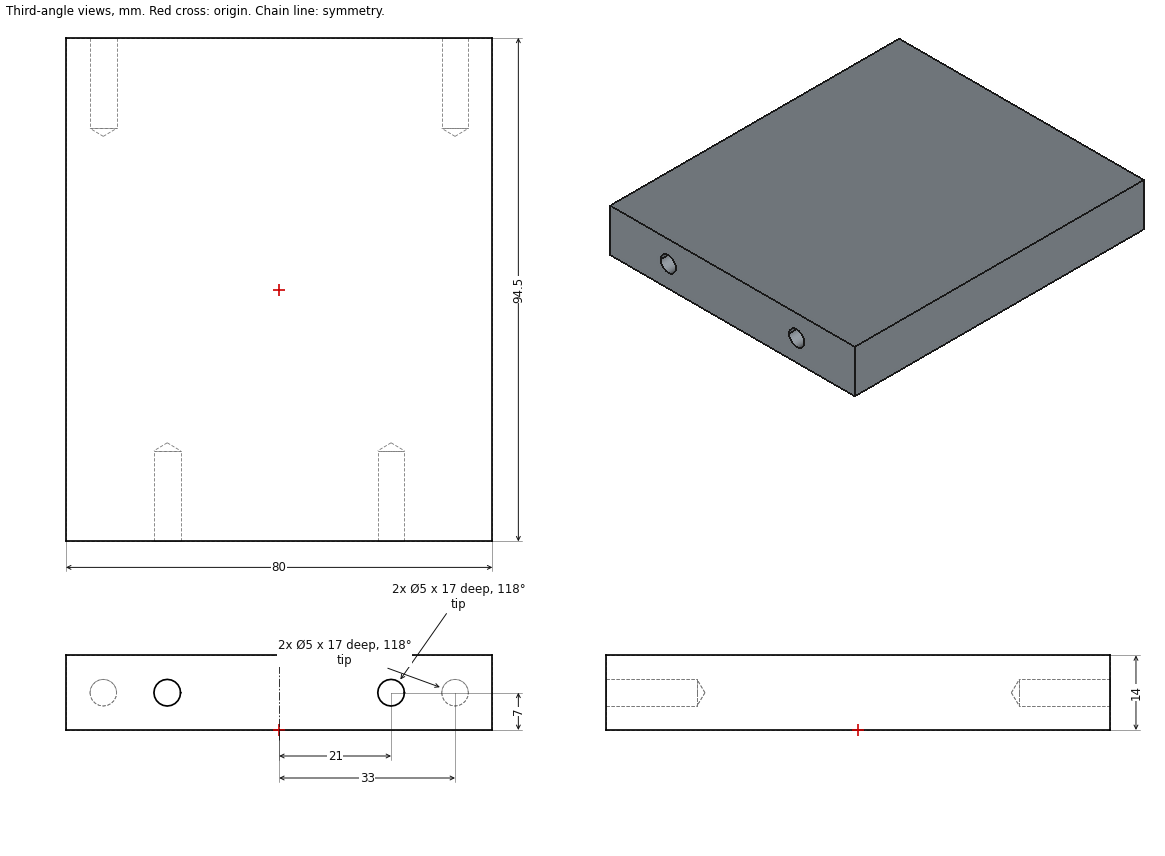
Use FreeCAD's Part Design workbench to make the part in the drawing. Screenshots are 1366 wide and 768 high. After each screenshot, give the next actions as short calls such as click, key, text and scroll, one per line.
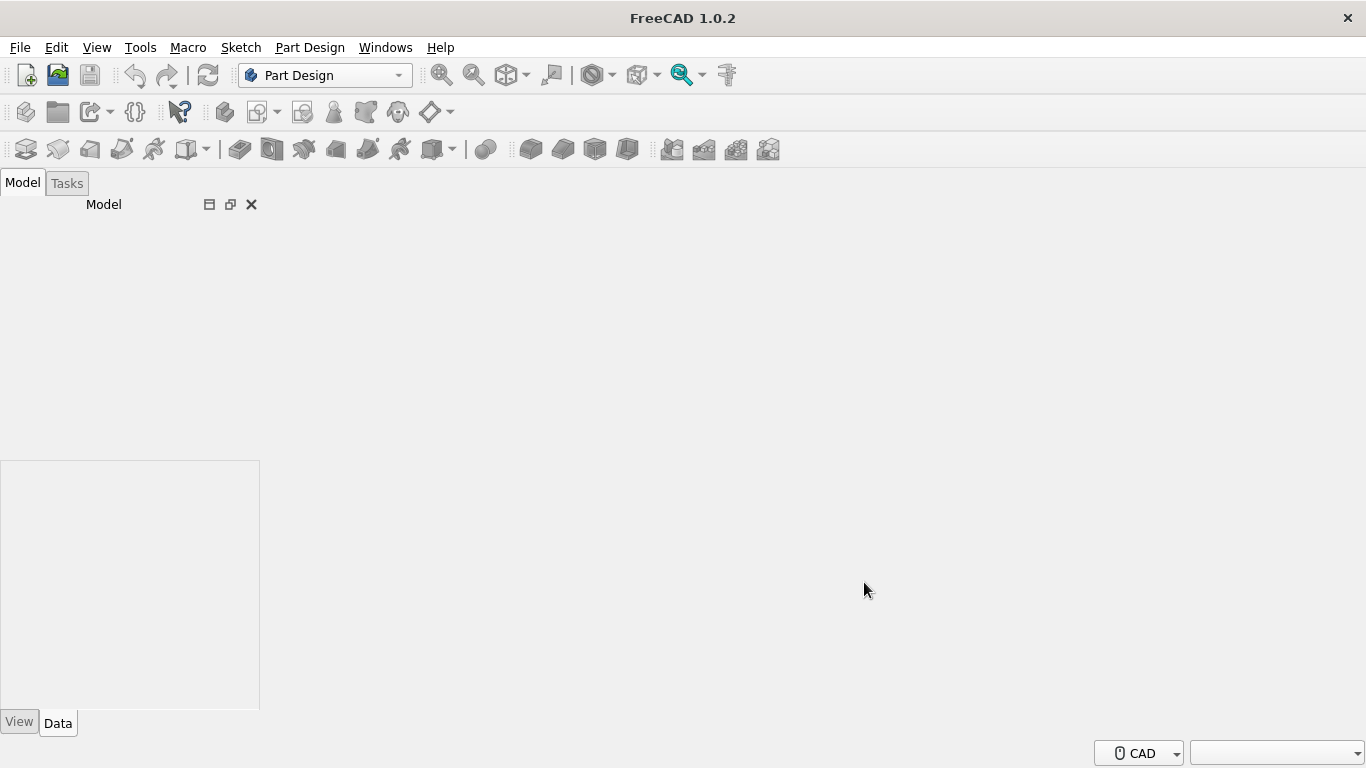
key(ctrl+n)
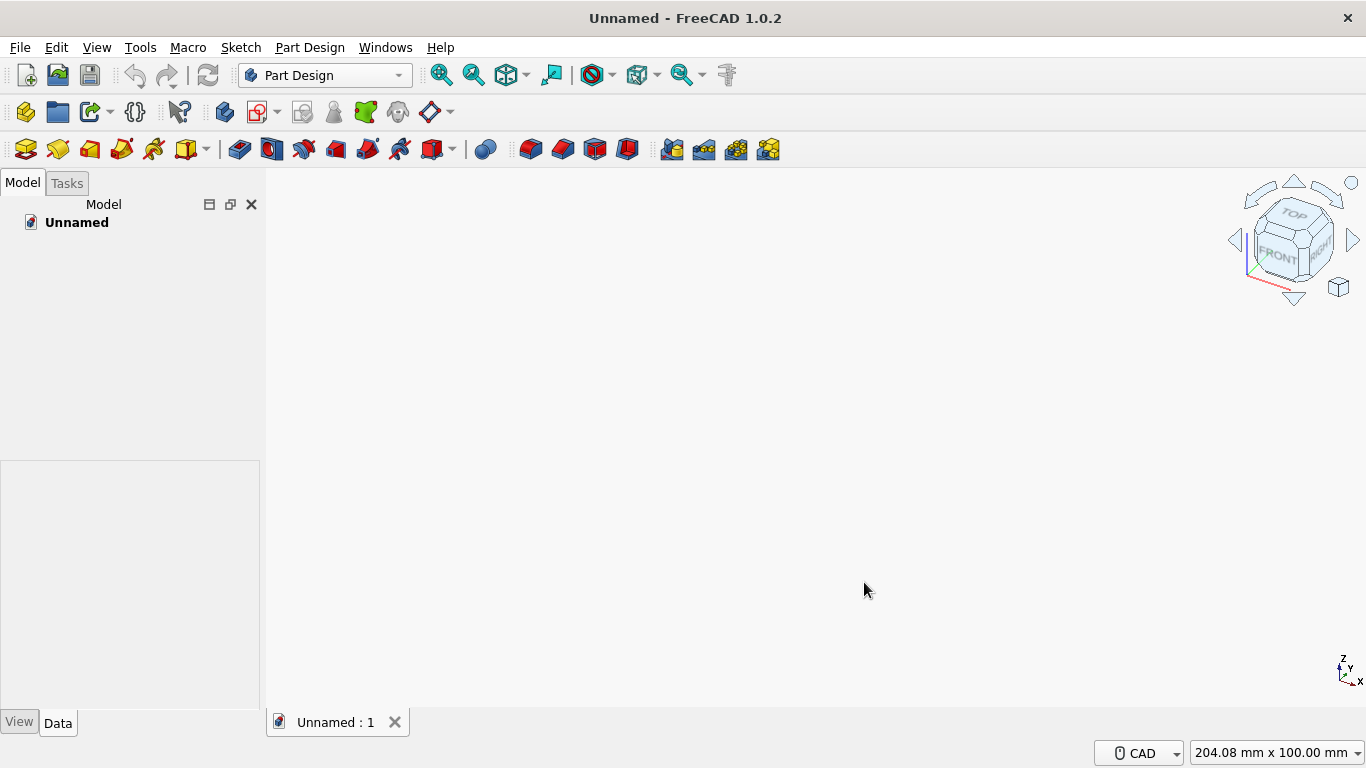
click(258, 112)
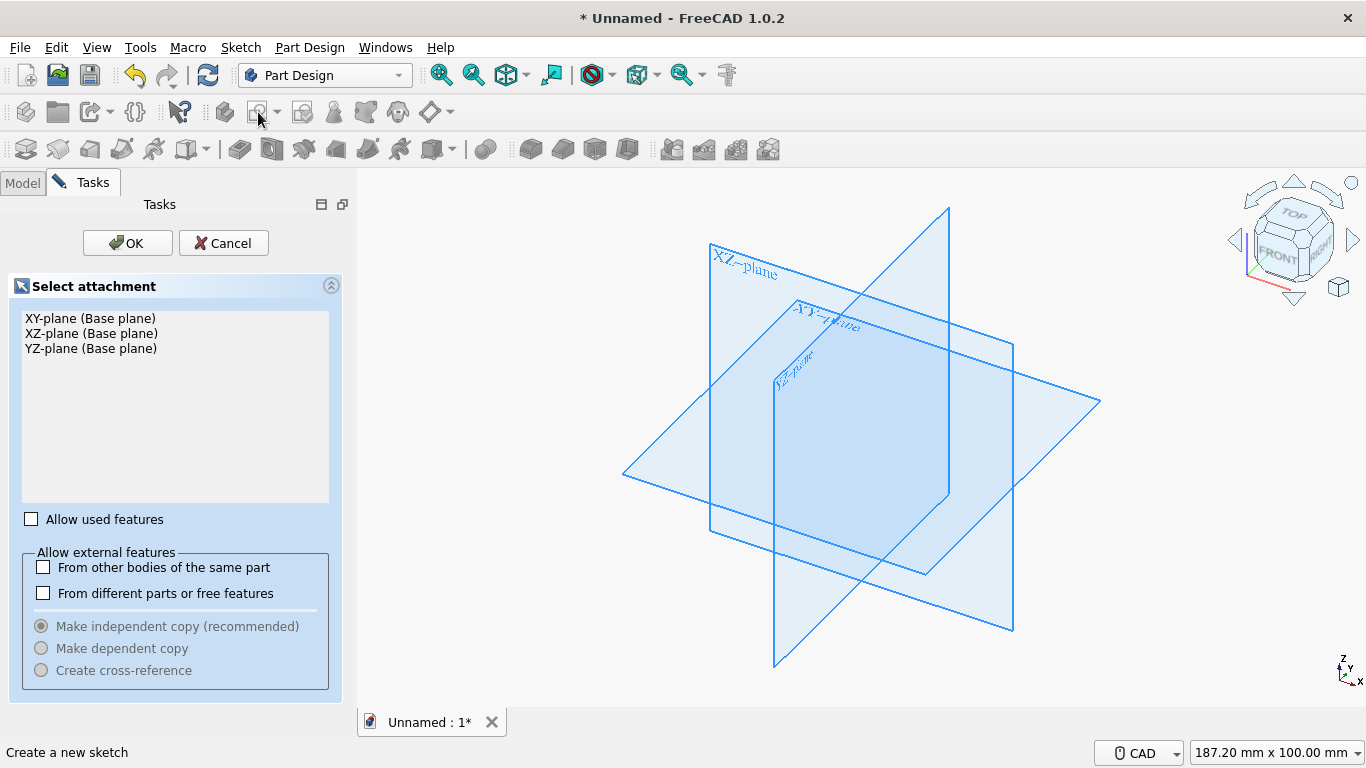
click(82, 318)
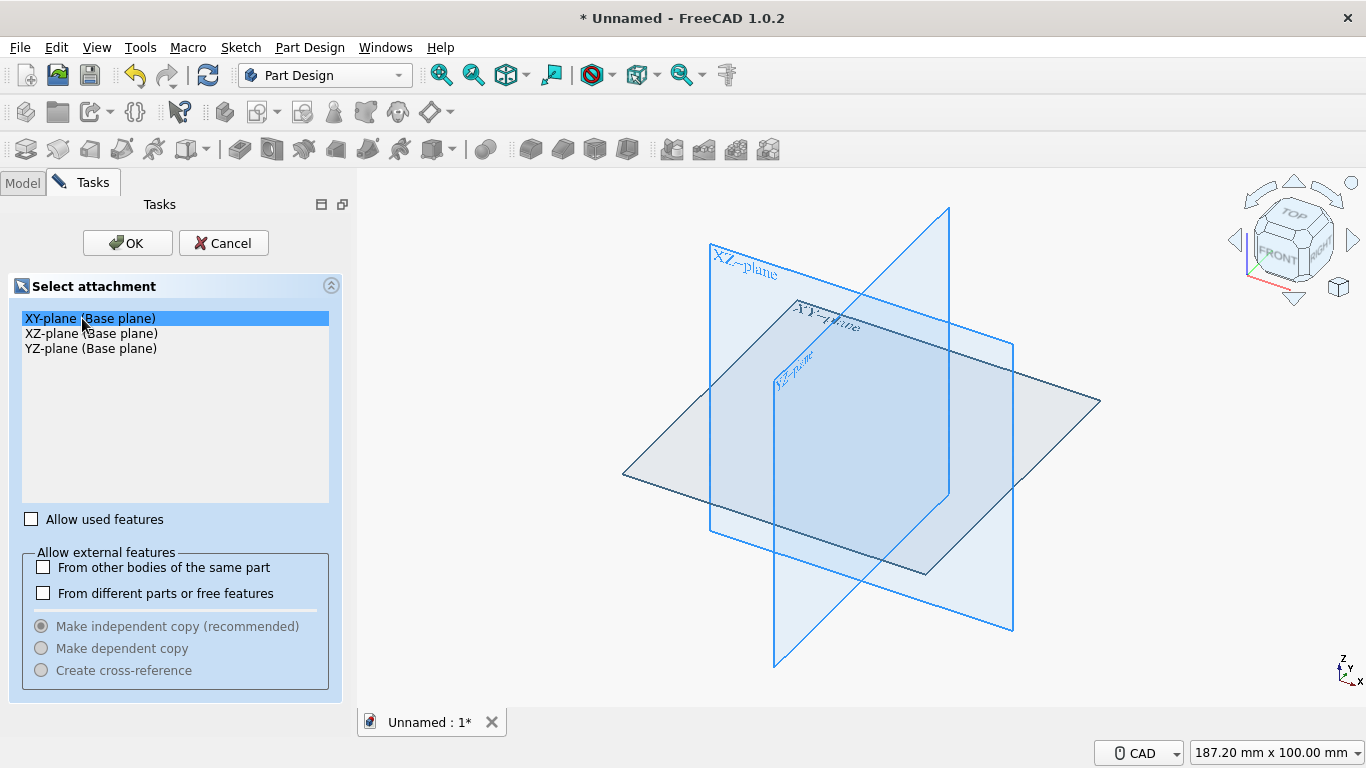
click(128, 243)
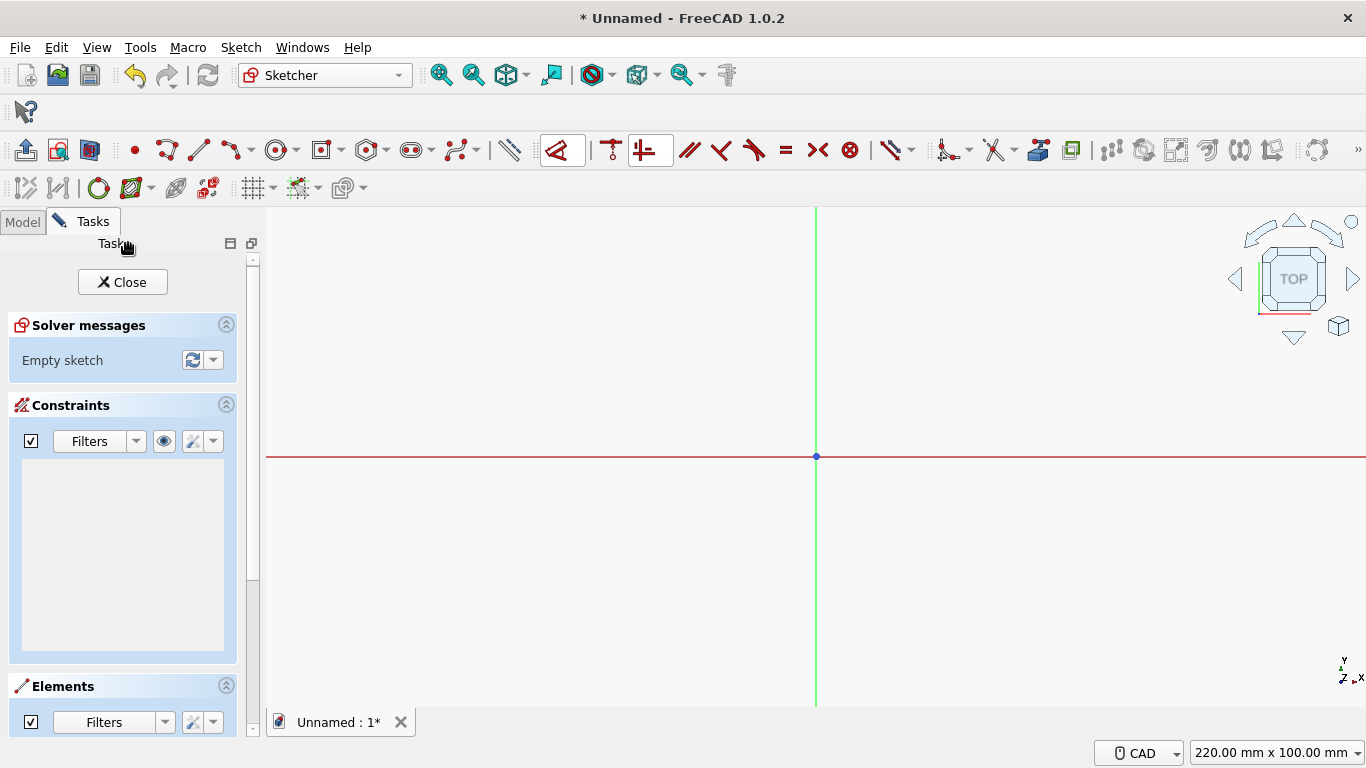
scroll(608, 457, down, 2)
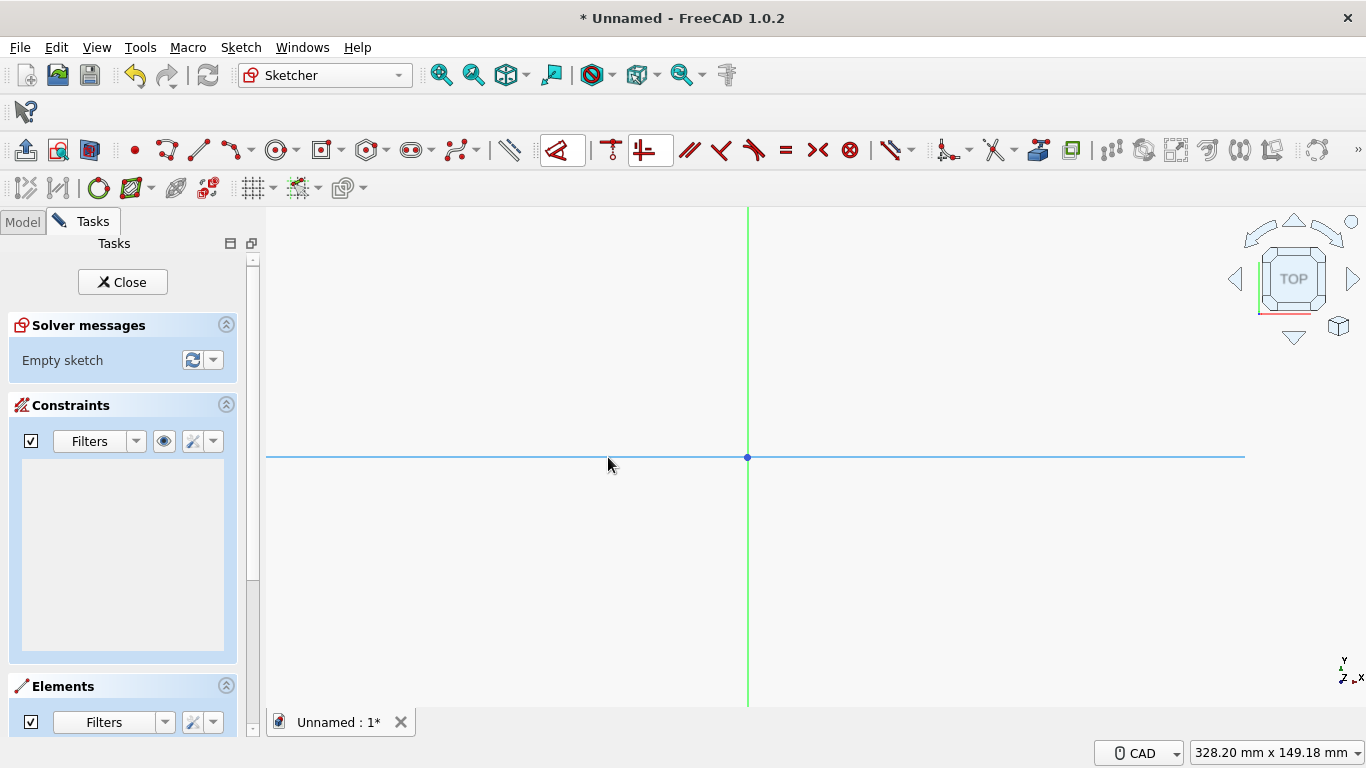
key(g)
key(v)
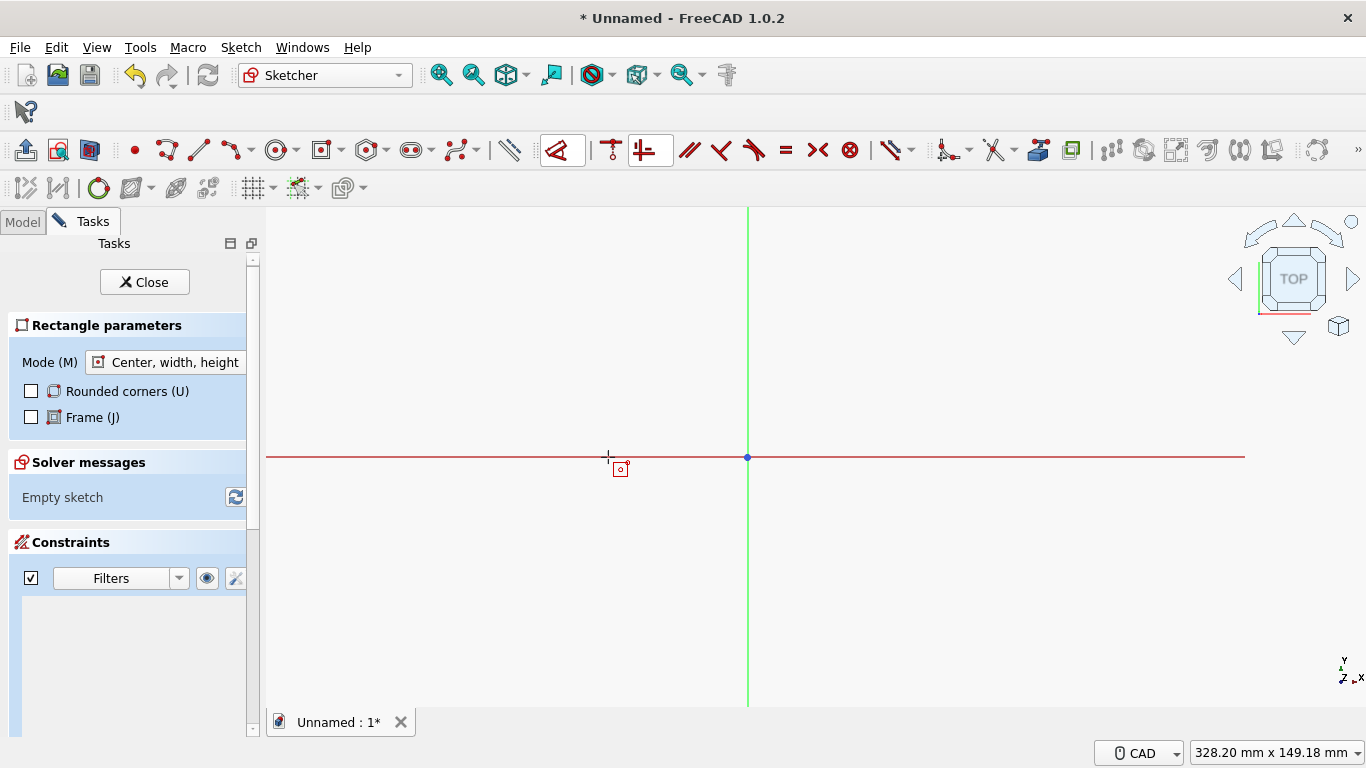
click(748, 457)
click(882, 299)
key(Escape)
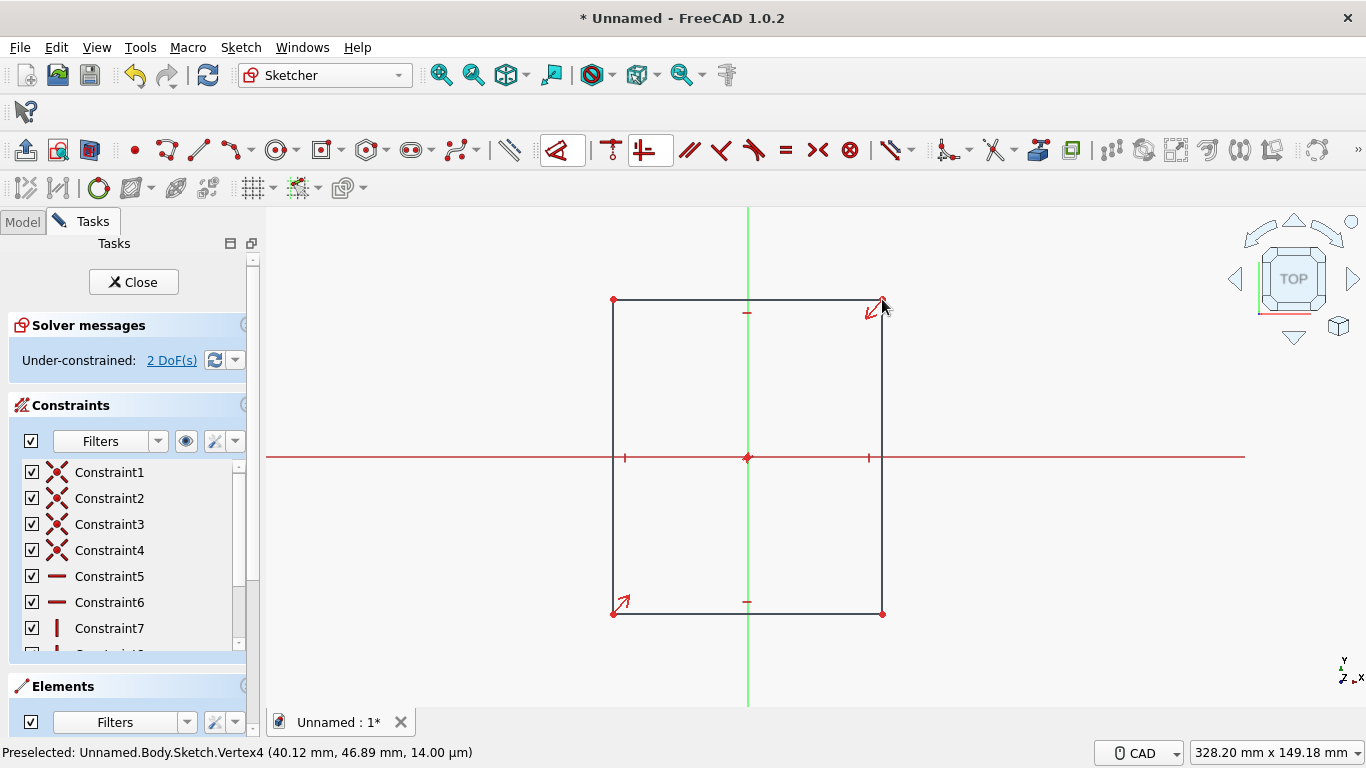
key(d)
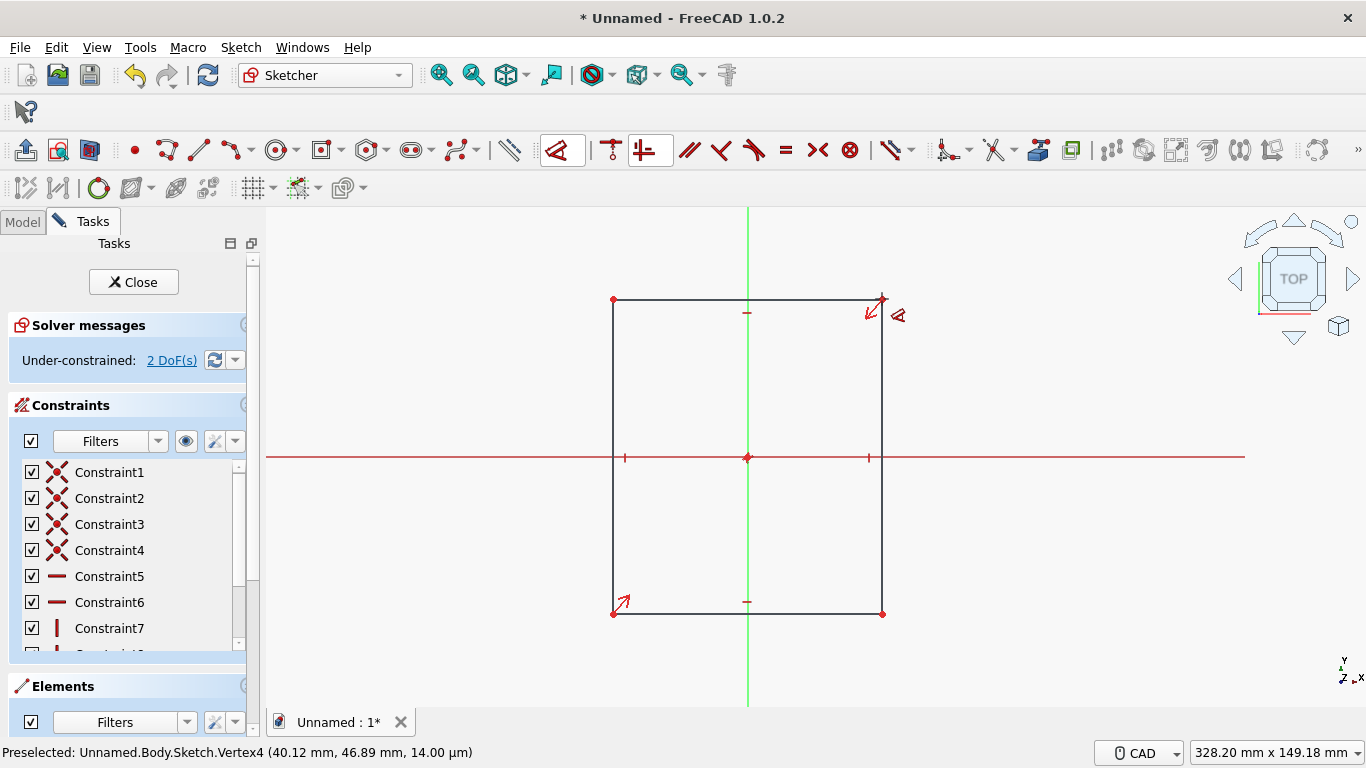
click(694, 614)
click(686, 648)